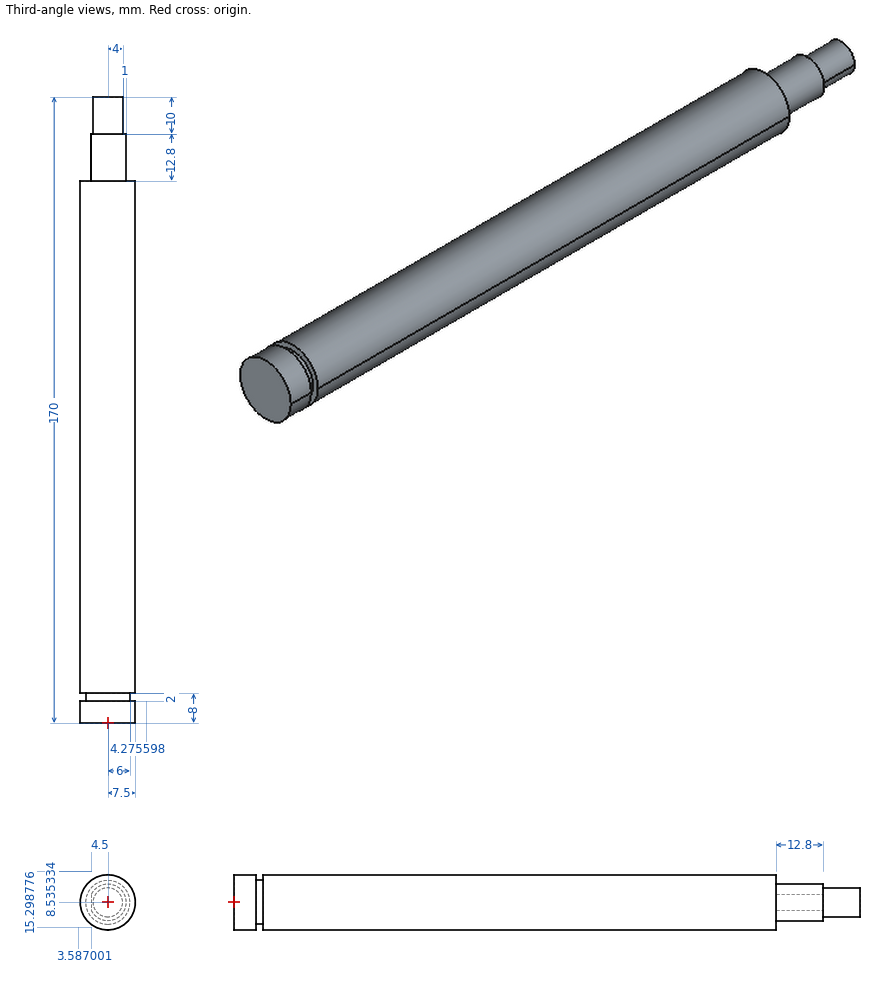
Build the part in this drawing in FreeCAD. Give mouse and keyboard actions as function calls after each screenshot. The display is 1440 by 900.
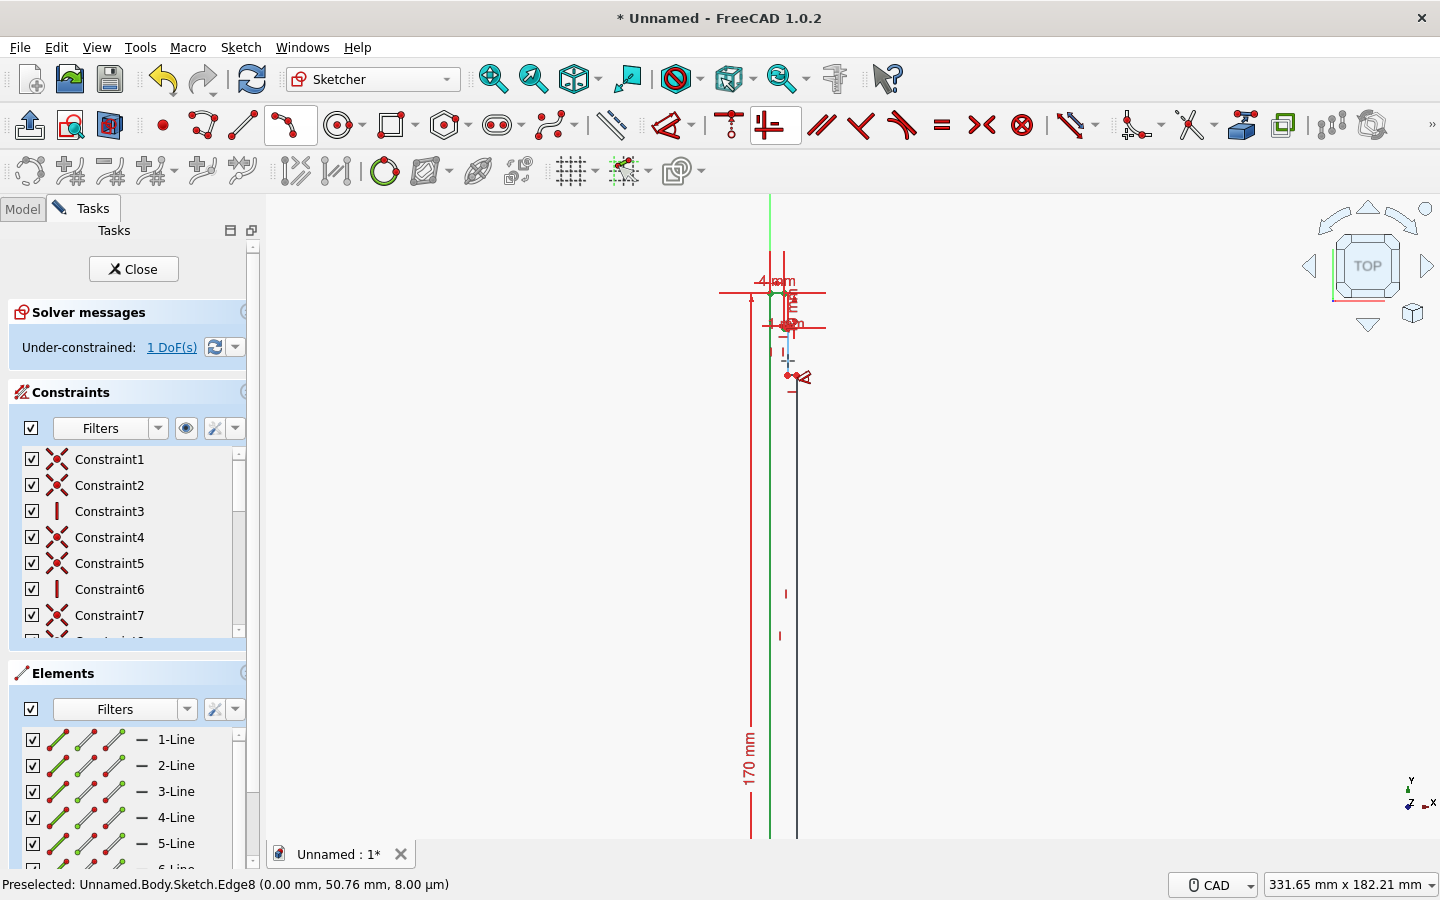
click(788, 361)
click(822, 352)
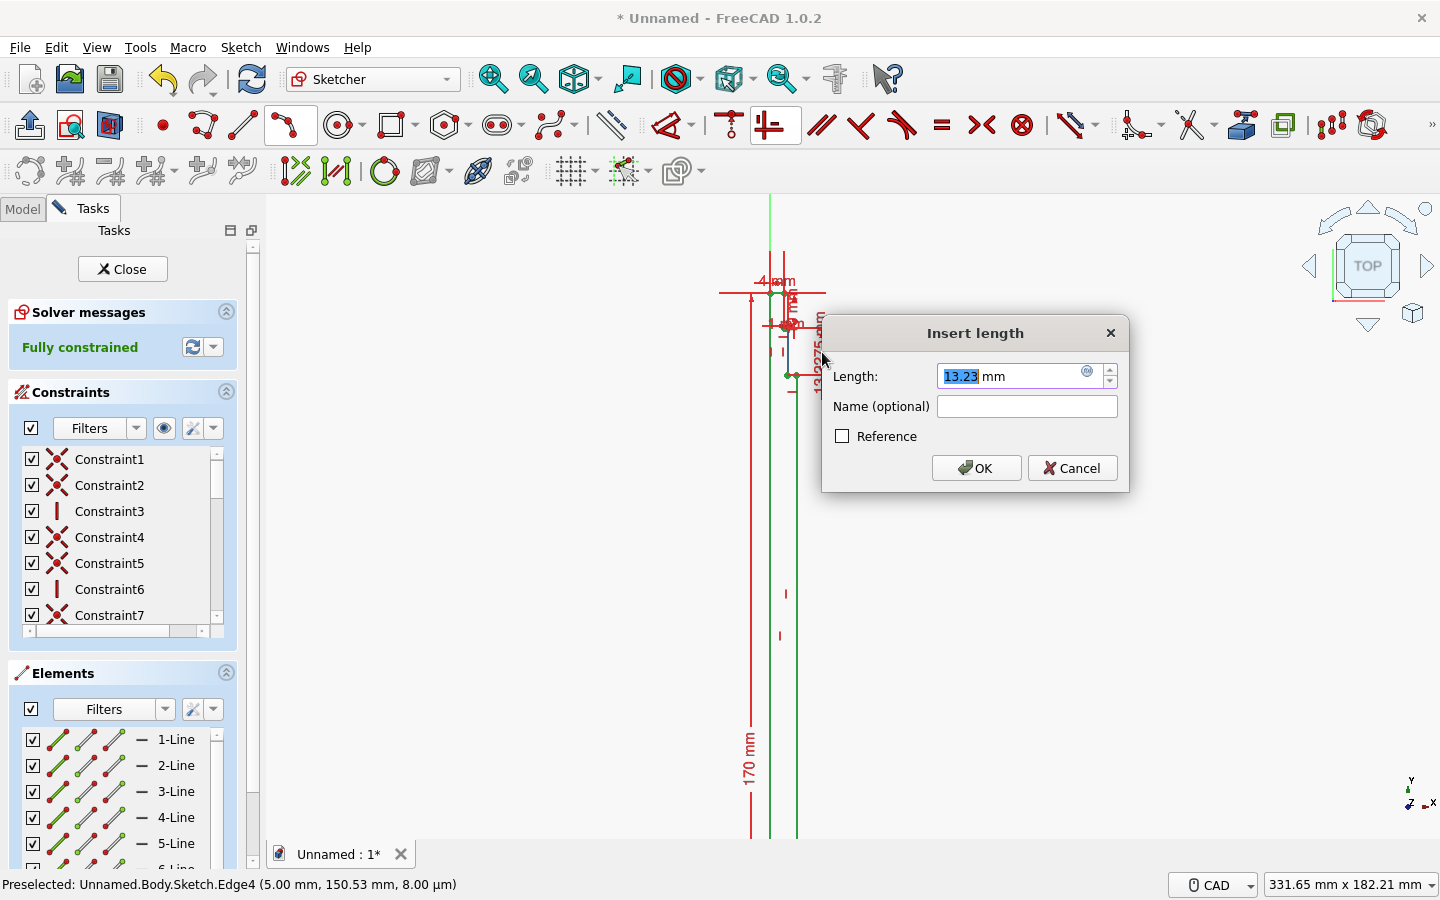
text(12.8)
key(Return)
key(Escape)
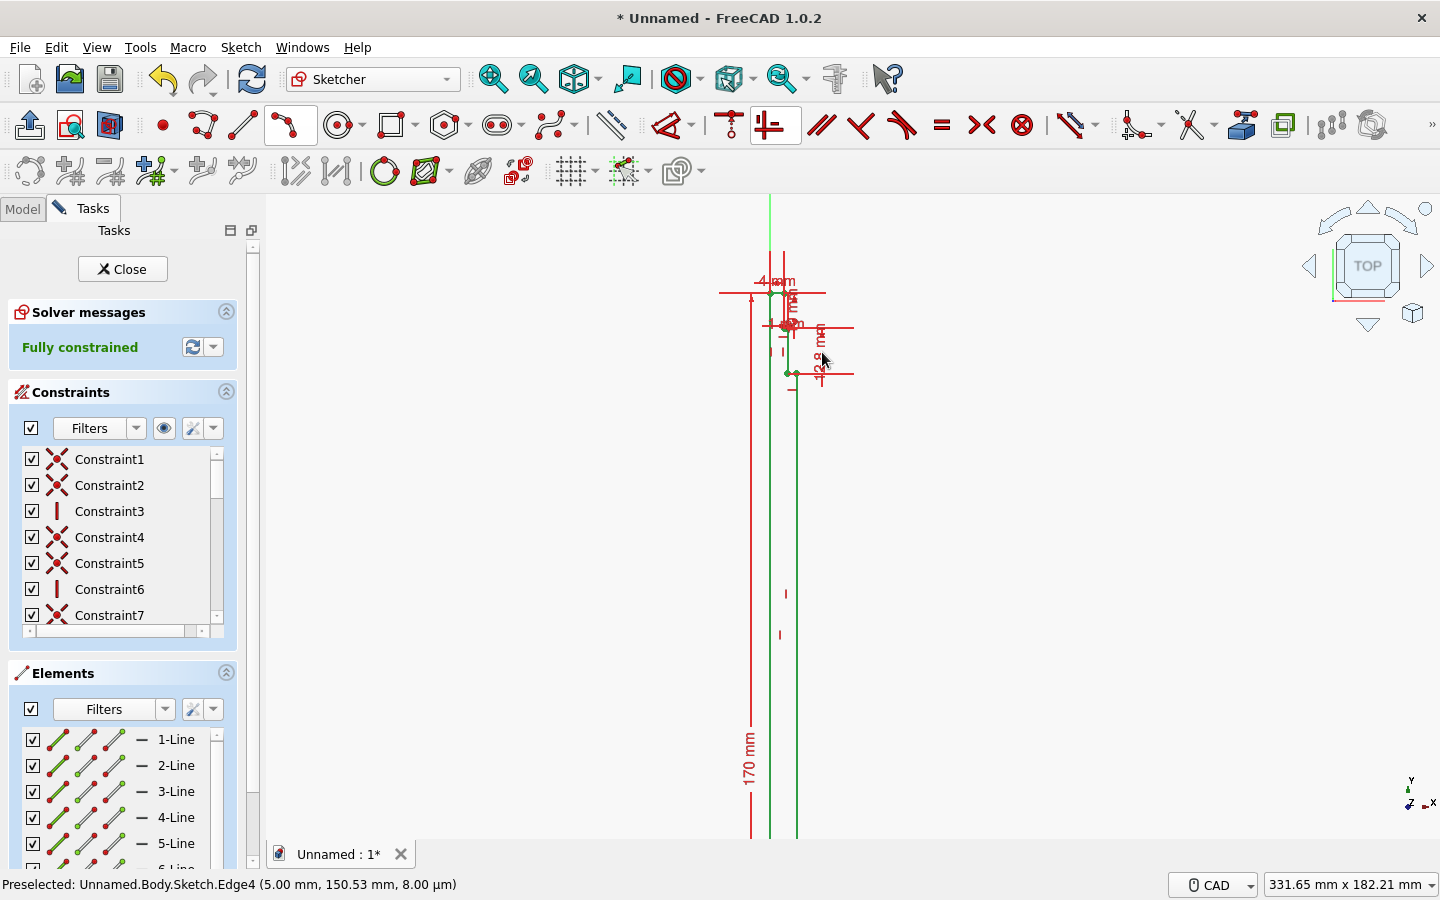
click(123, 269)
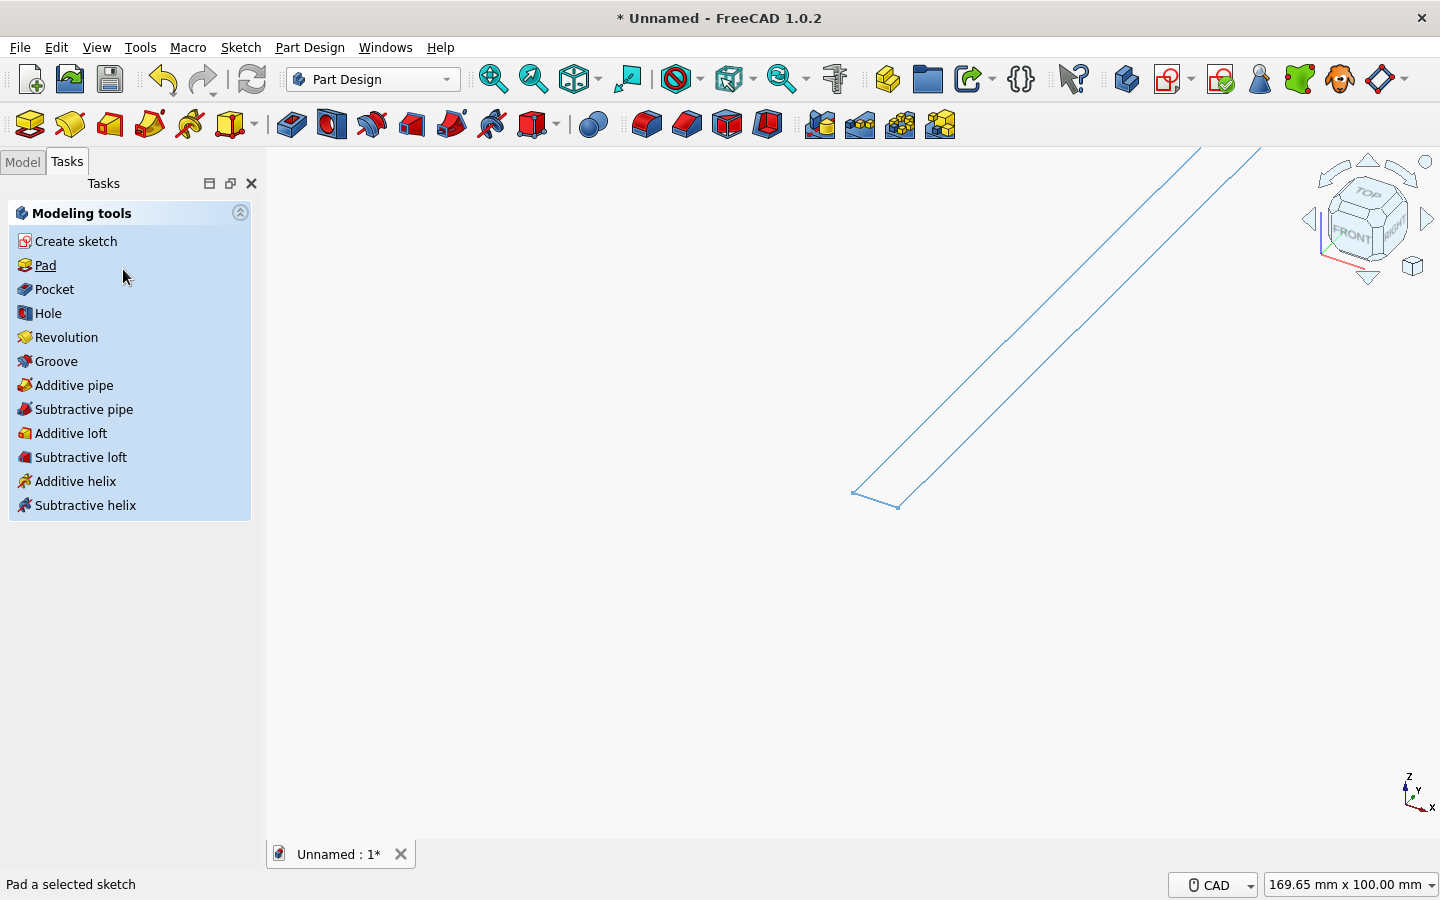
click(70, 124)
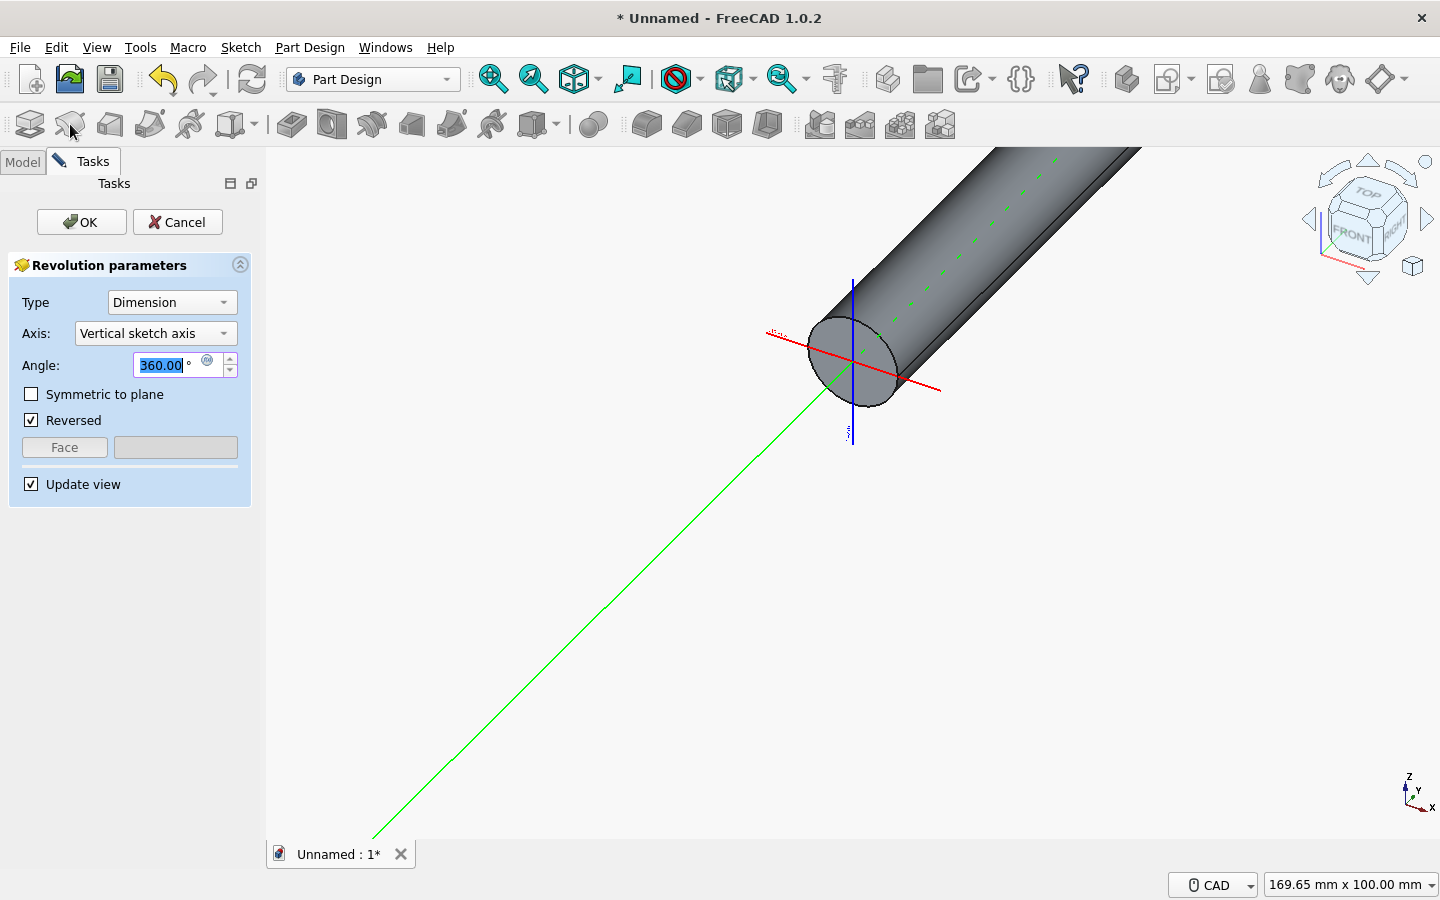
click(82, 222)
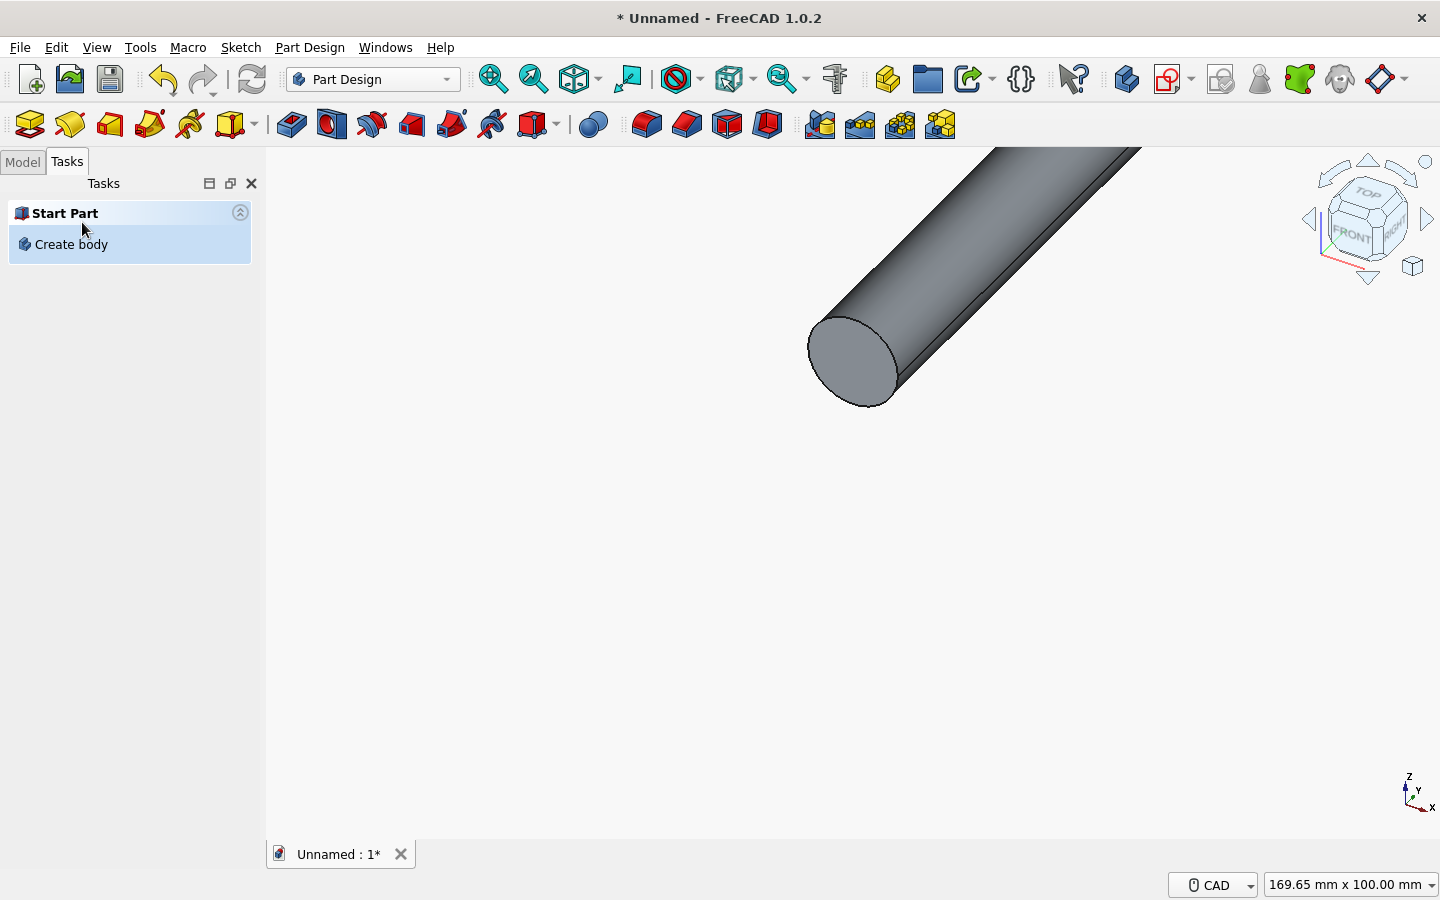
click(494, 80)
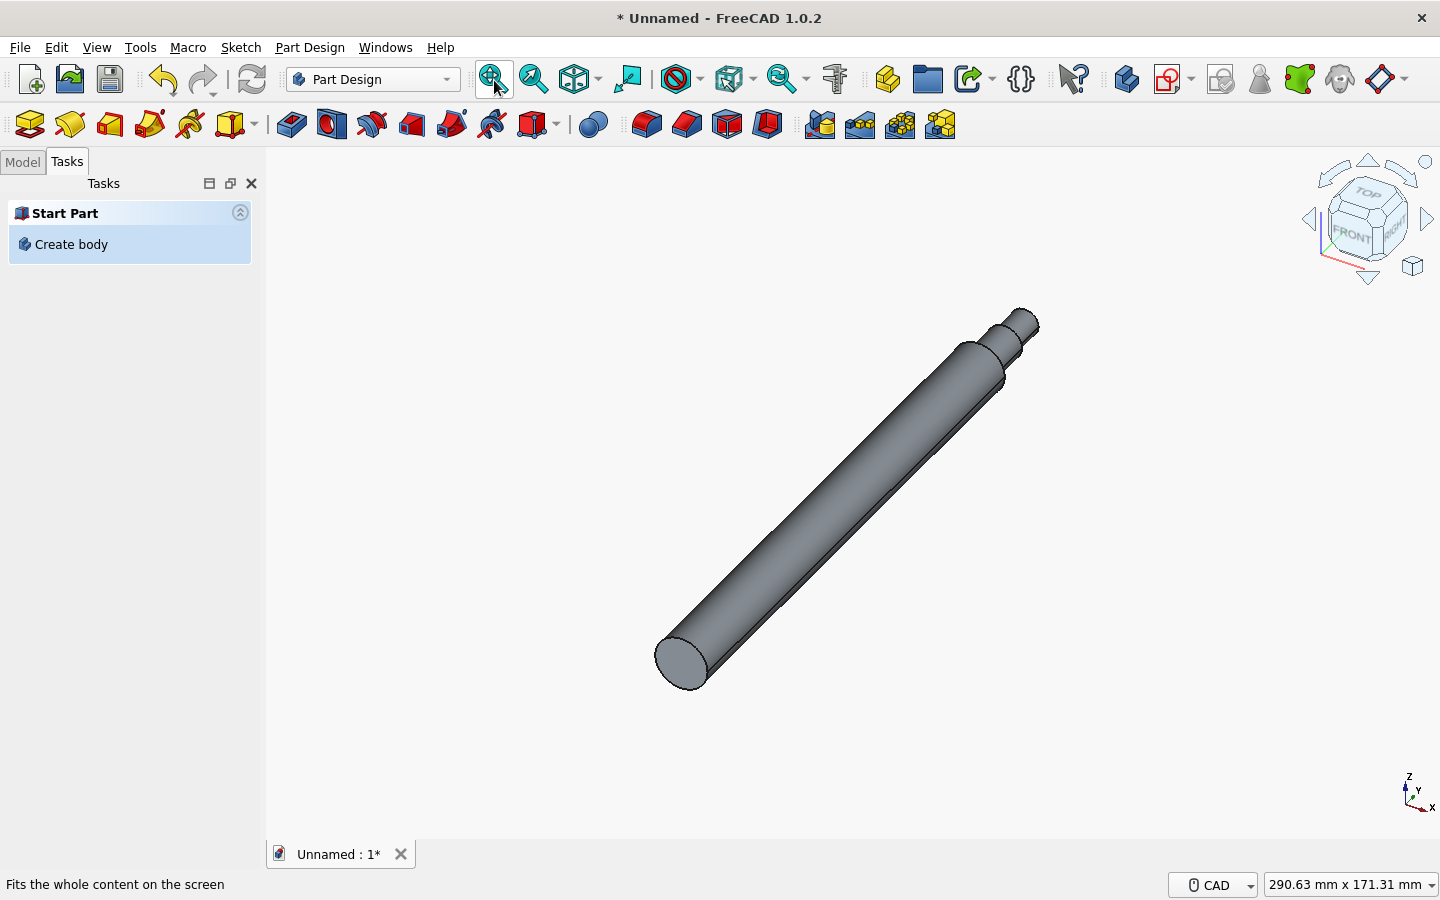
key(4)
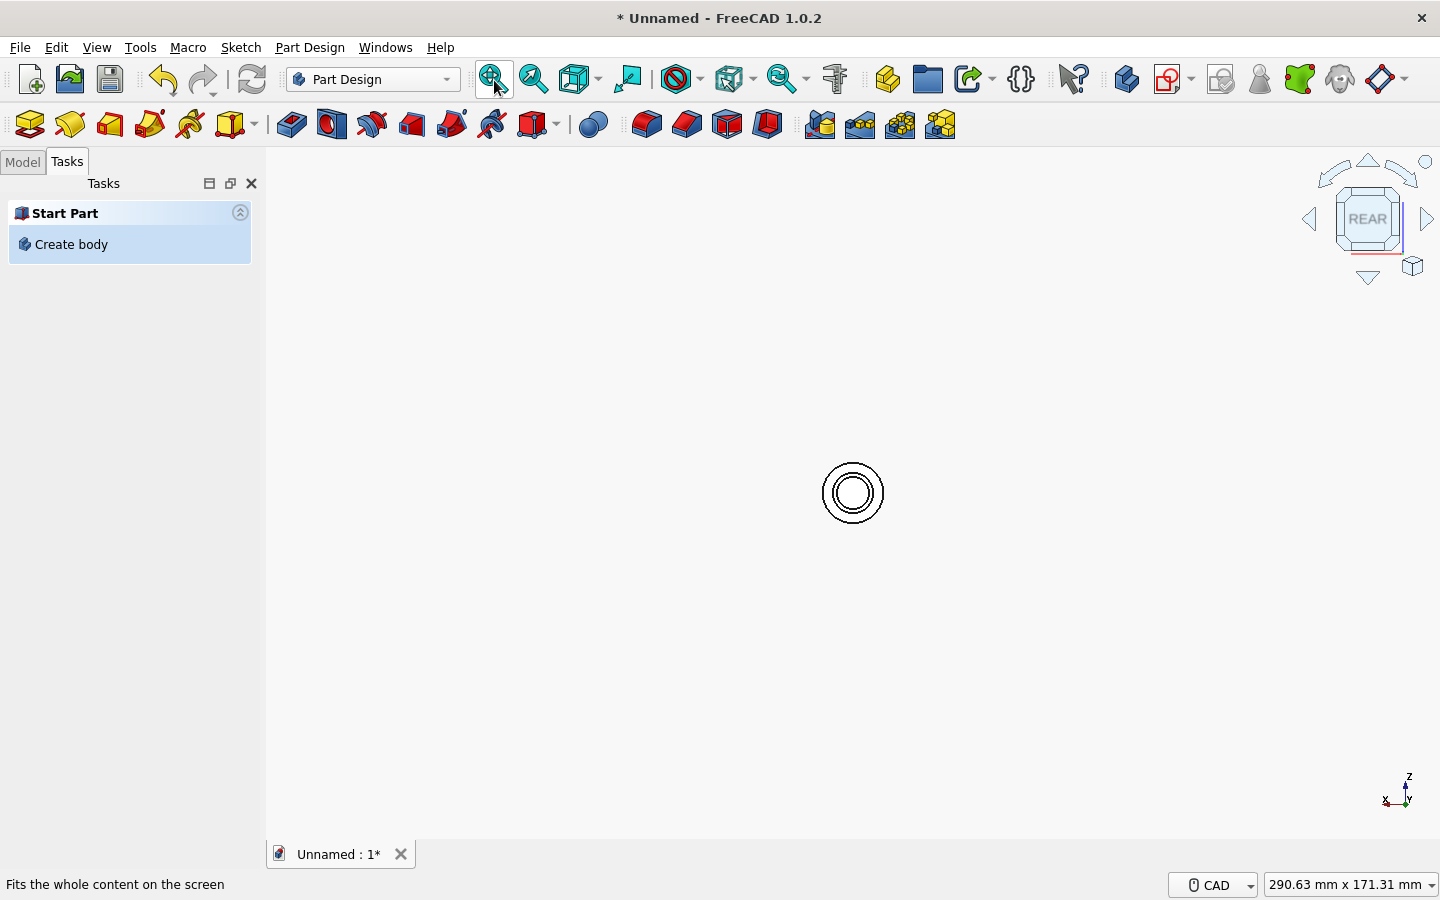
click(494, 80)